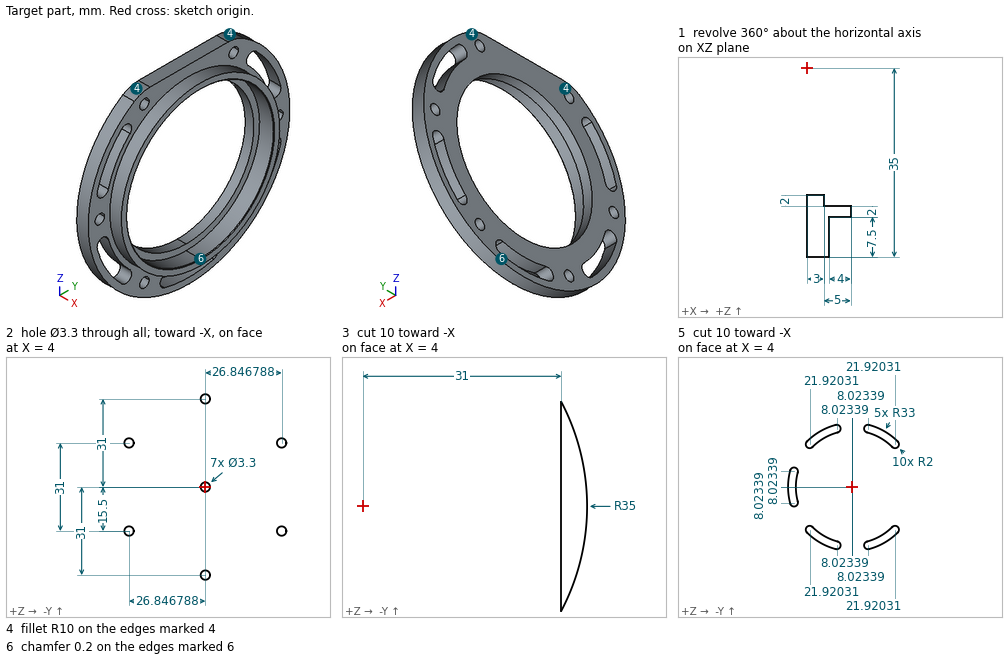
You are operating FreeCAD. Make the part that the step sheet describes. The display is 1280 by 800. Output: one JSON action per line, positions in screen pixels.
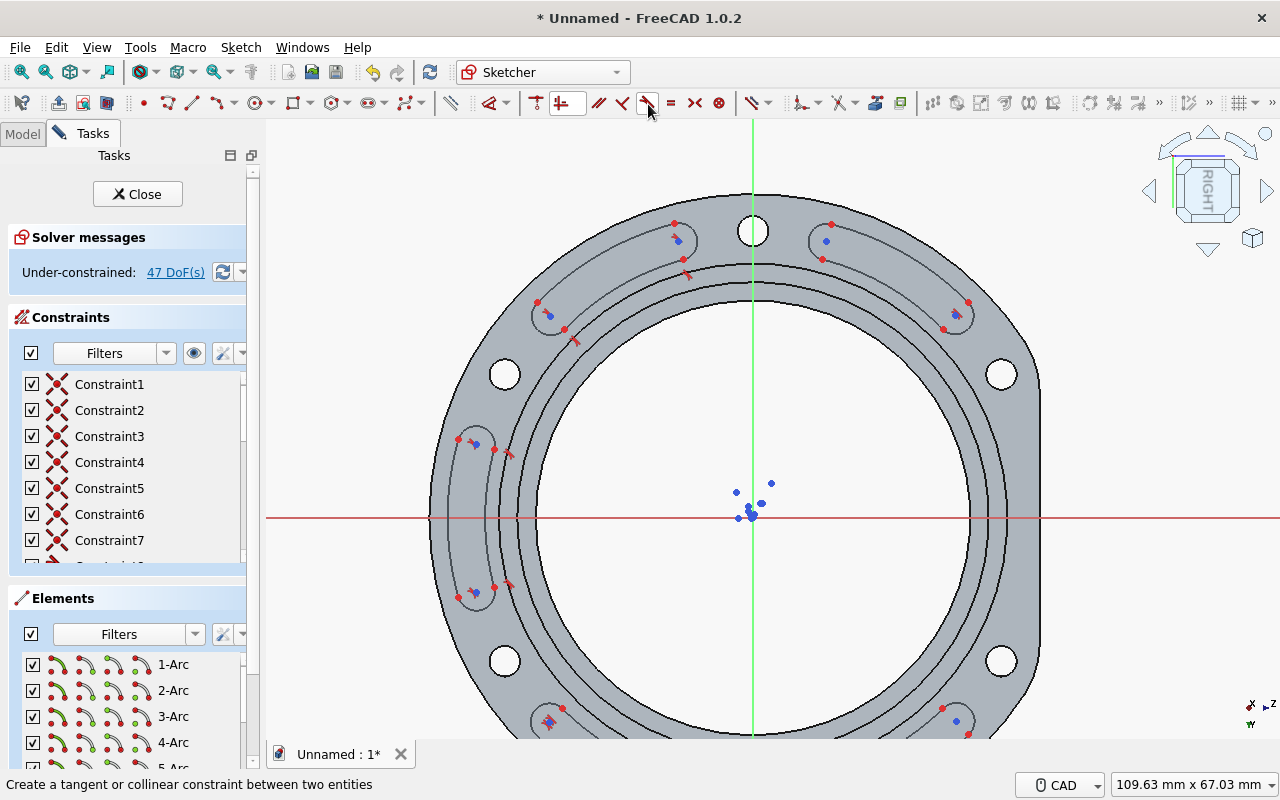
{"action": "left_click", "coordinate": [959, 334]}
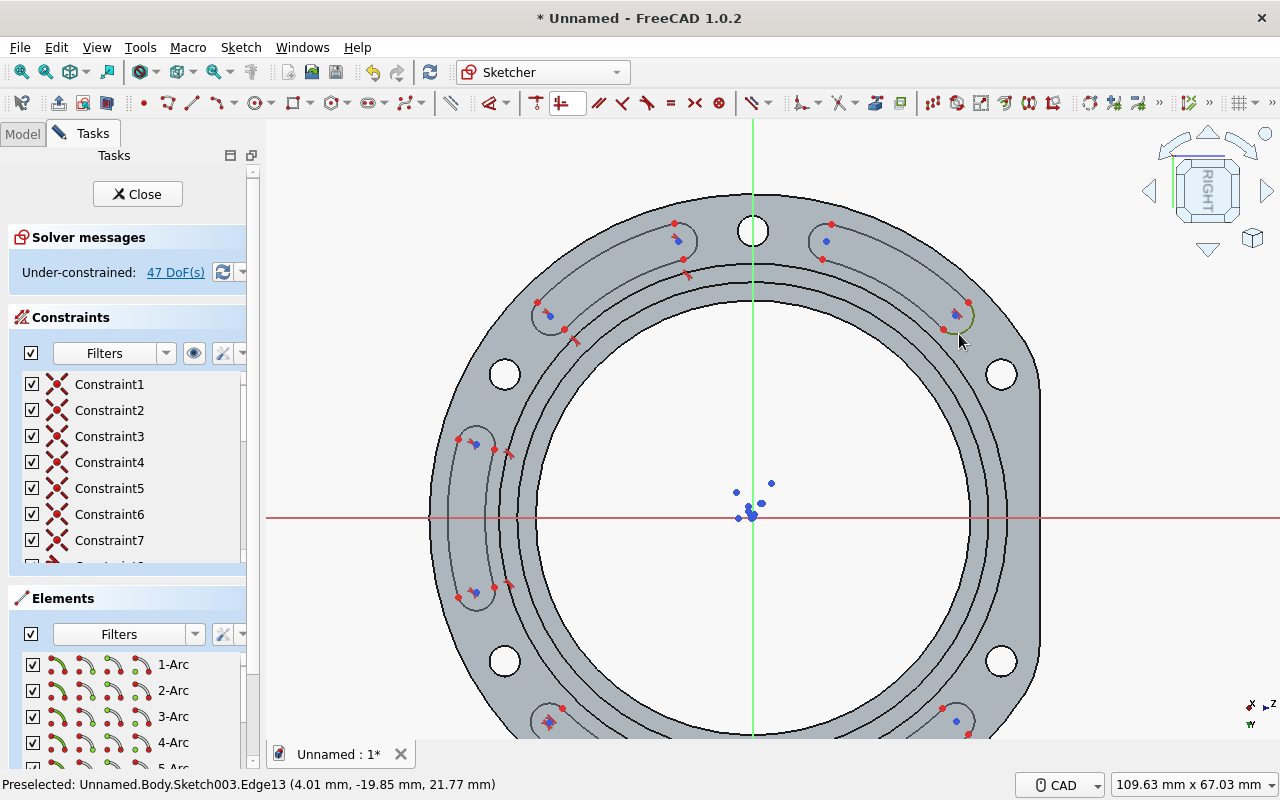
{"action": "left_click", "coordinate": [911, 302]}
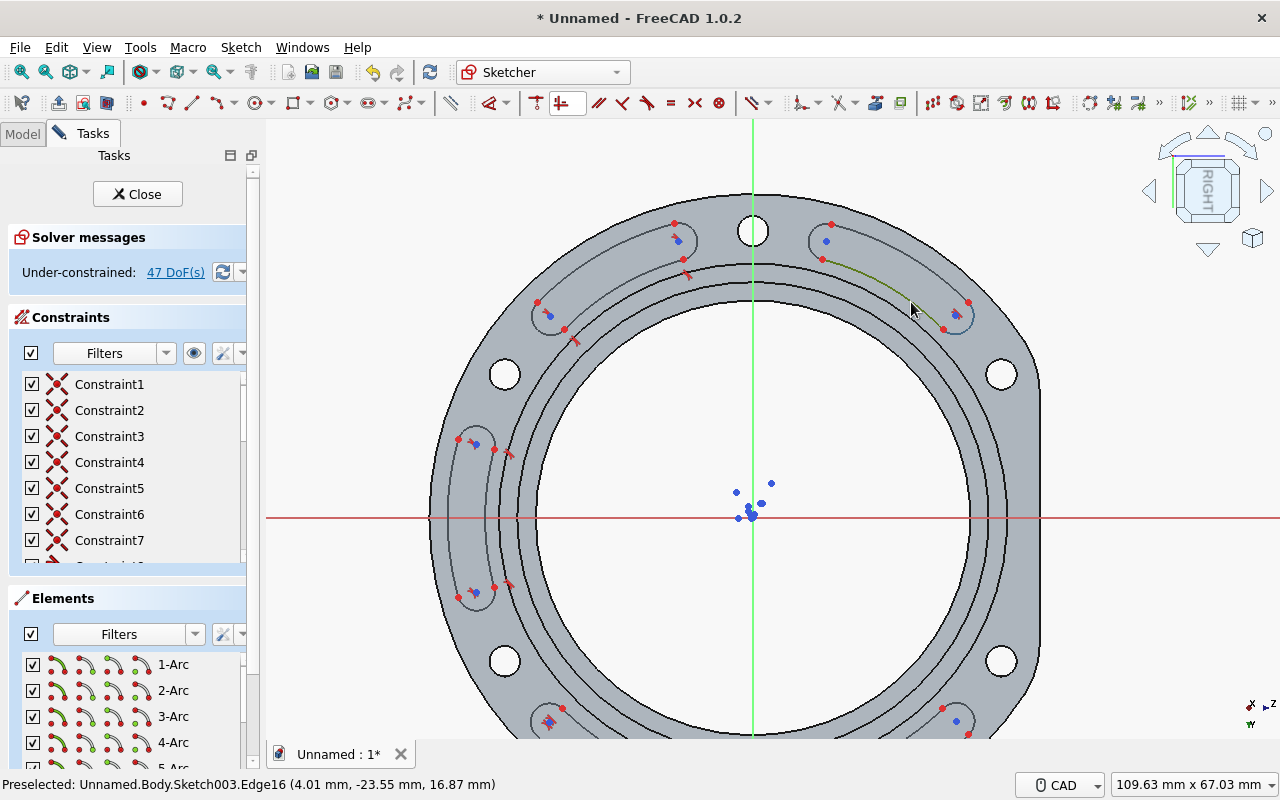
{"action": "left_click", "coordinate": [648, 104]}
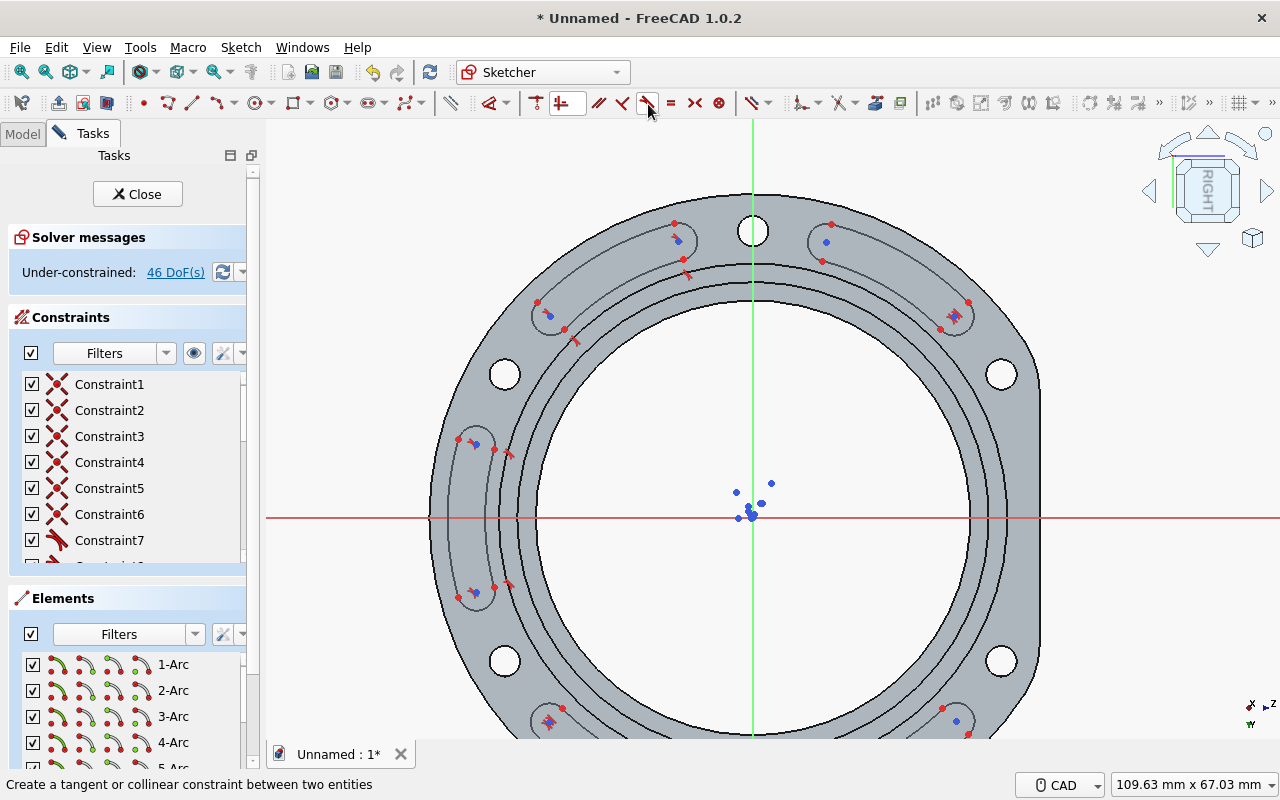
{"action": "left_click", "coordinate": [932, 272]}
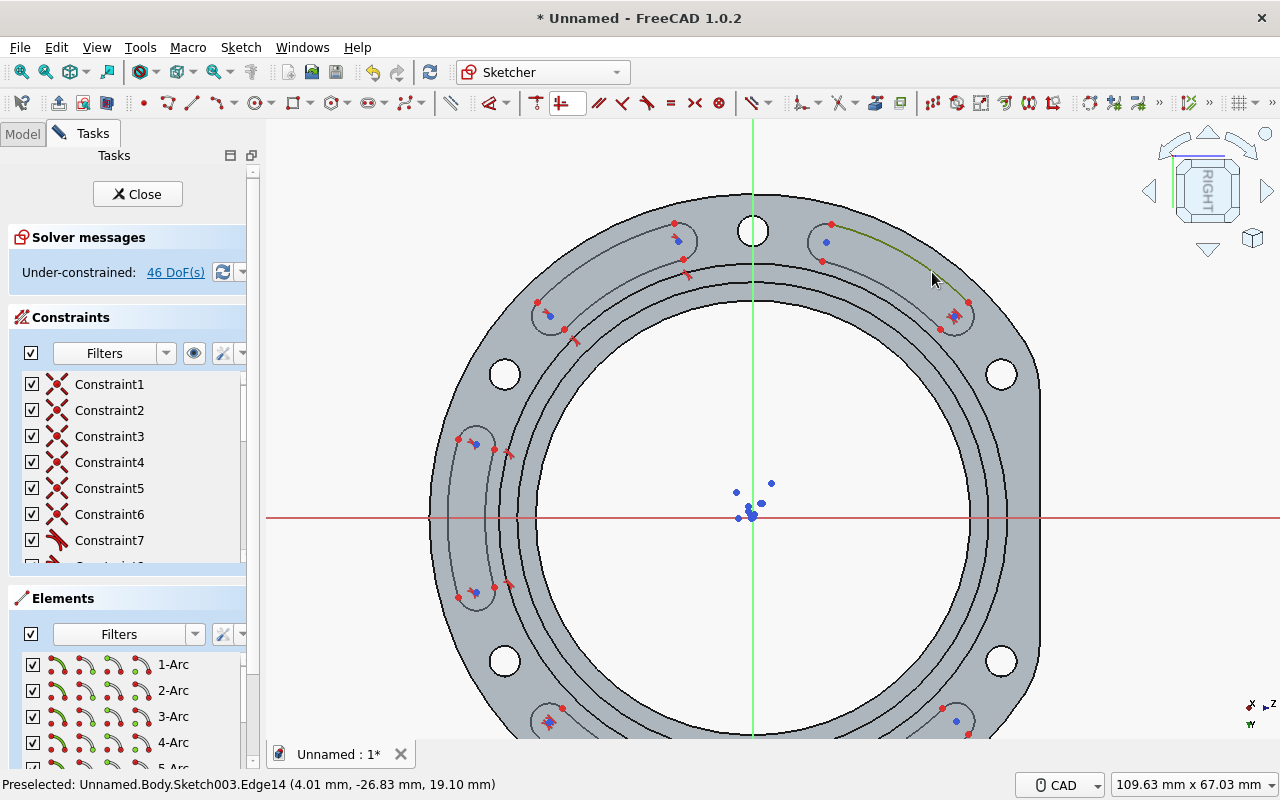
{"action": "left_click", "coordinate": [815, 228]}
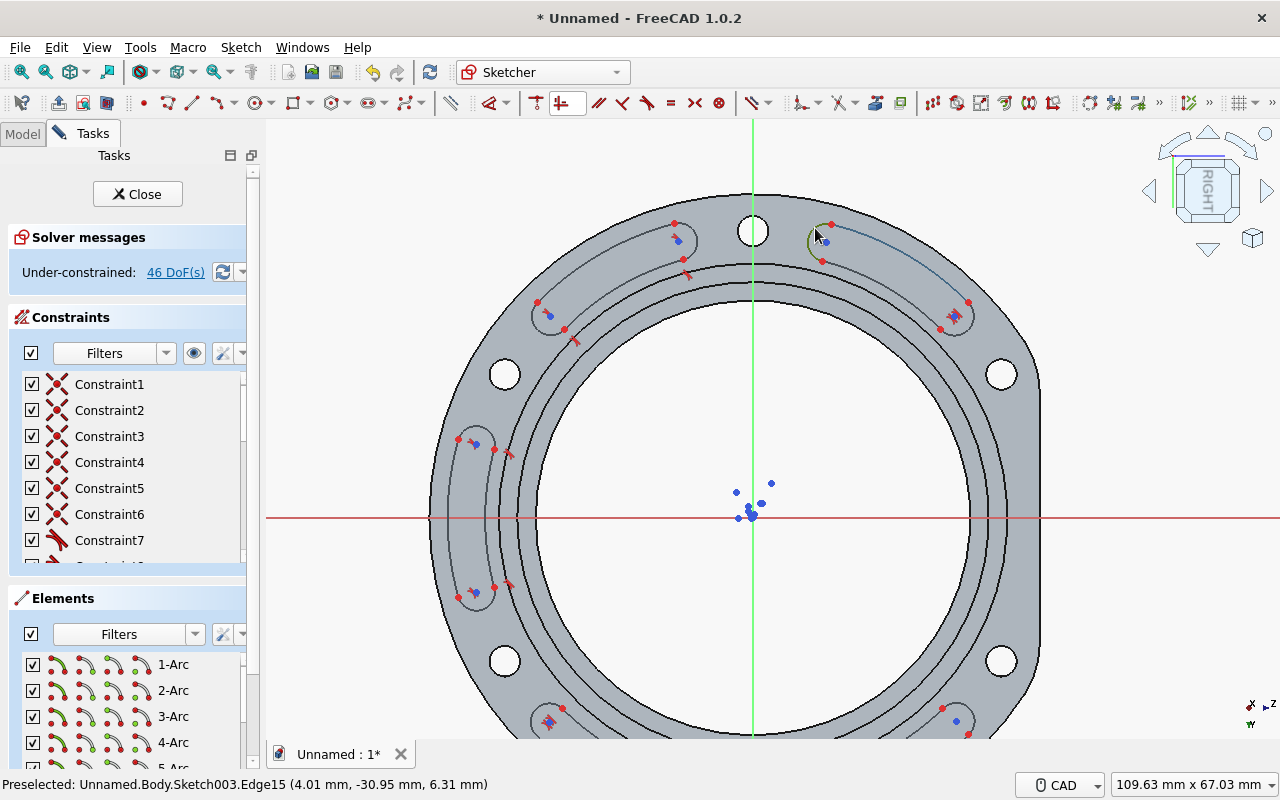
{"action": "left_click", "coordinate": [648, 104]}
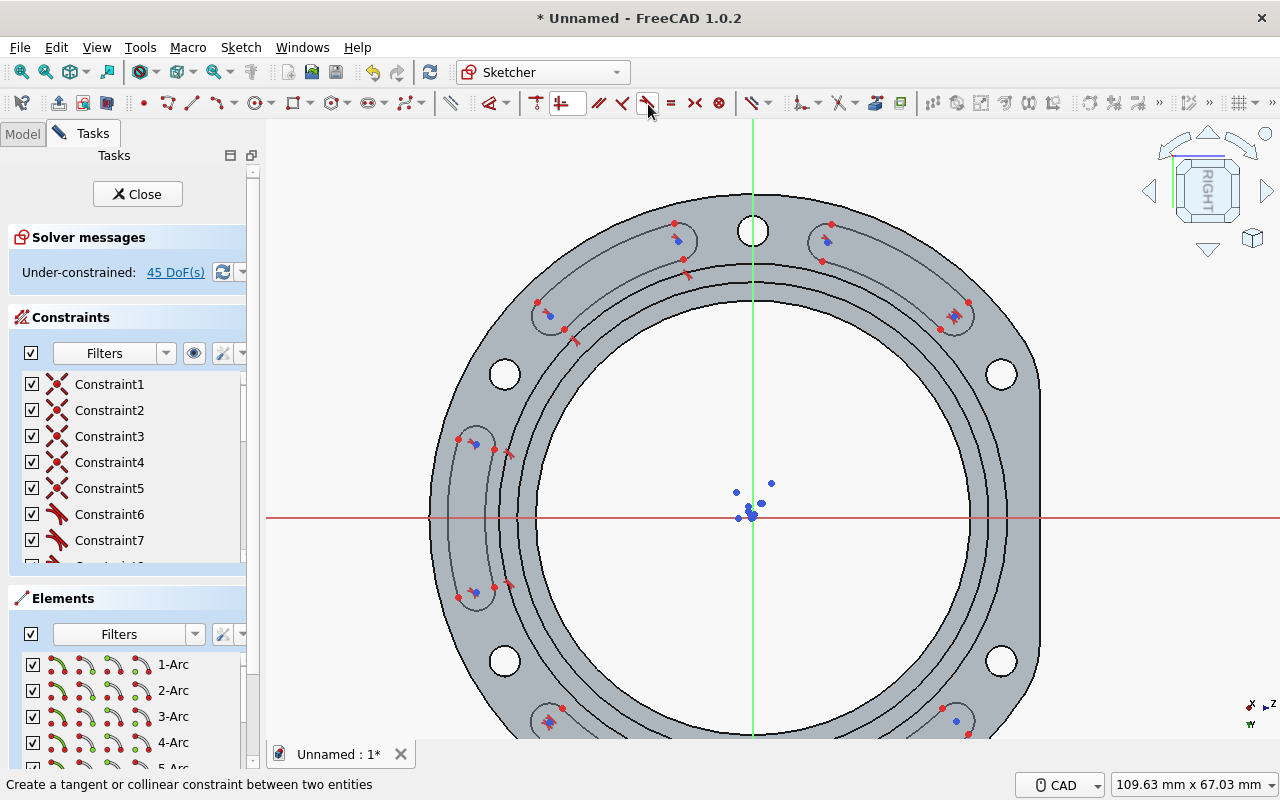
{"action": "left_click", "coordinate": [815, 228]}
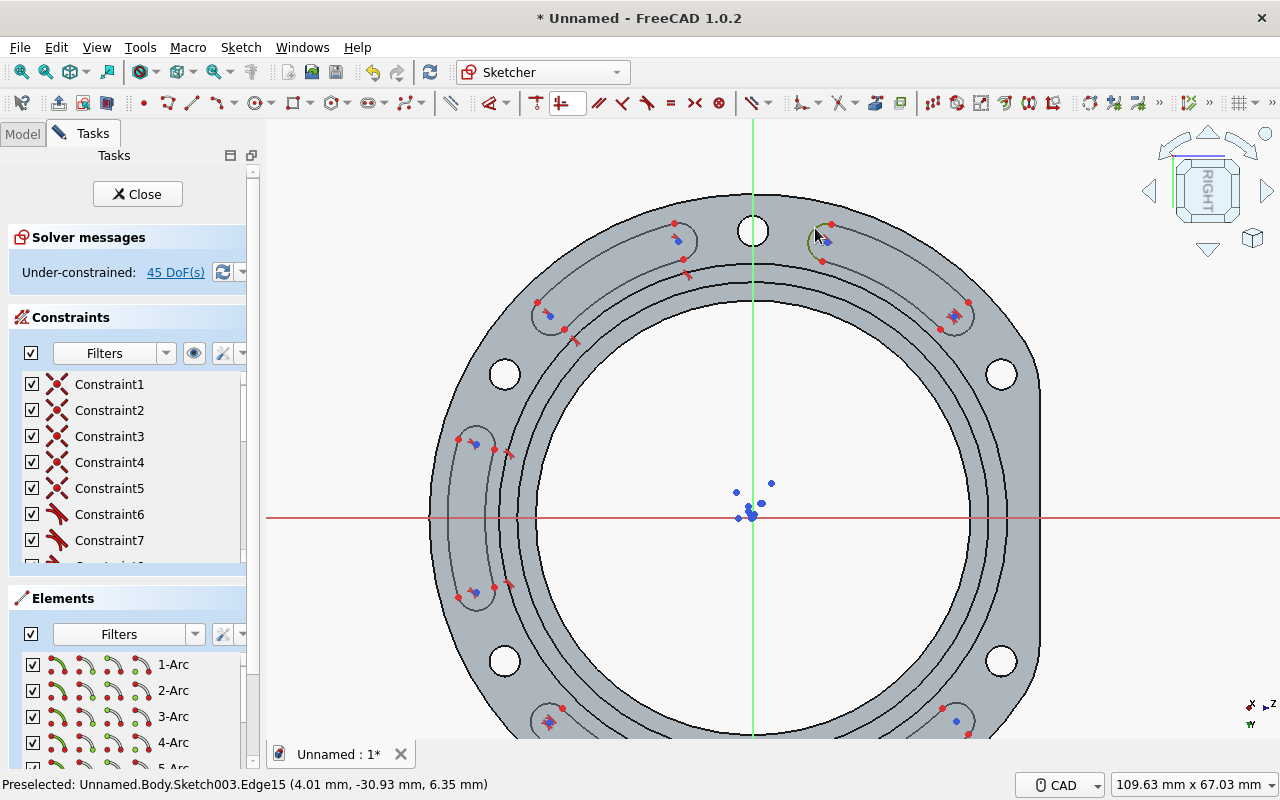
{"action": "left_click", "coordinate": [910, 302]}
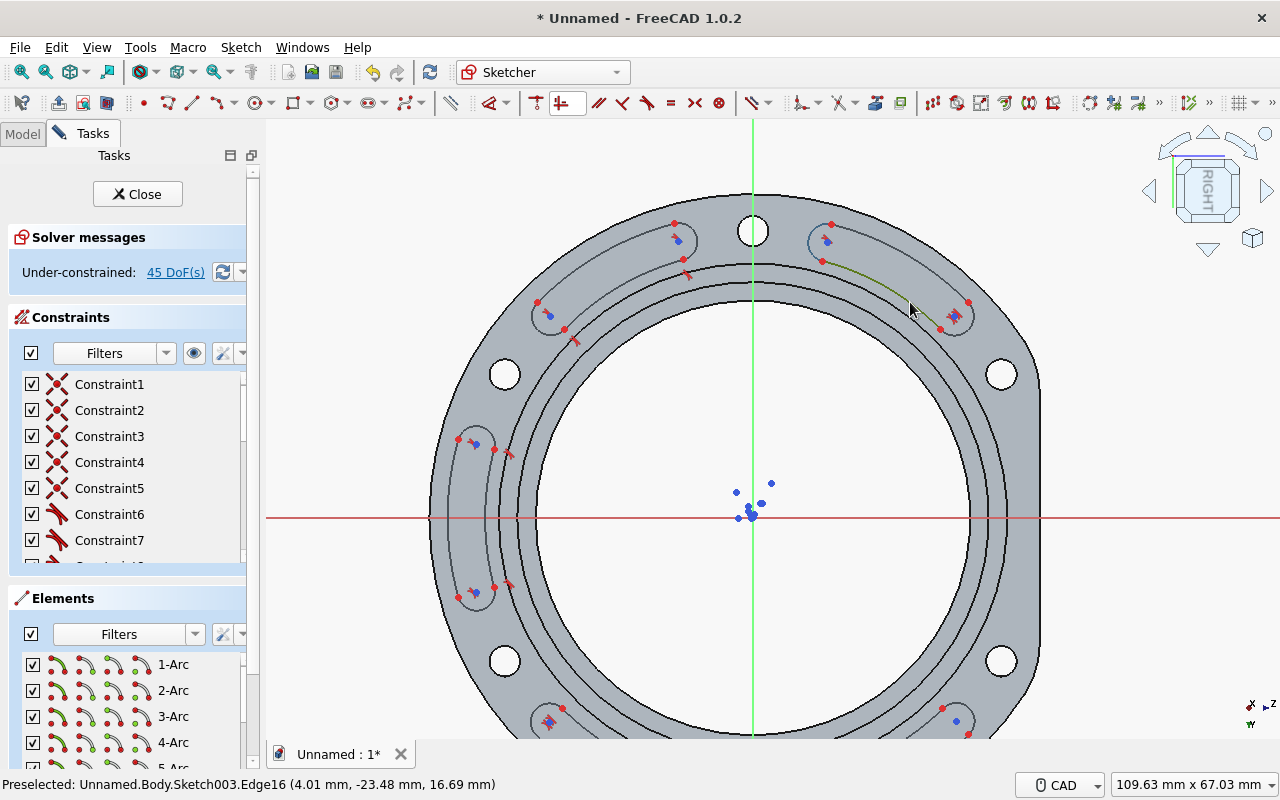
{"action": "left_click", "coordinate": [648, 104]}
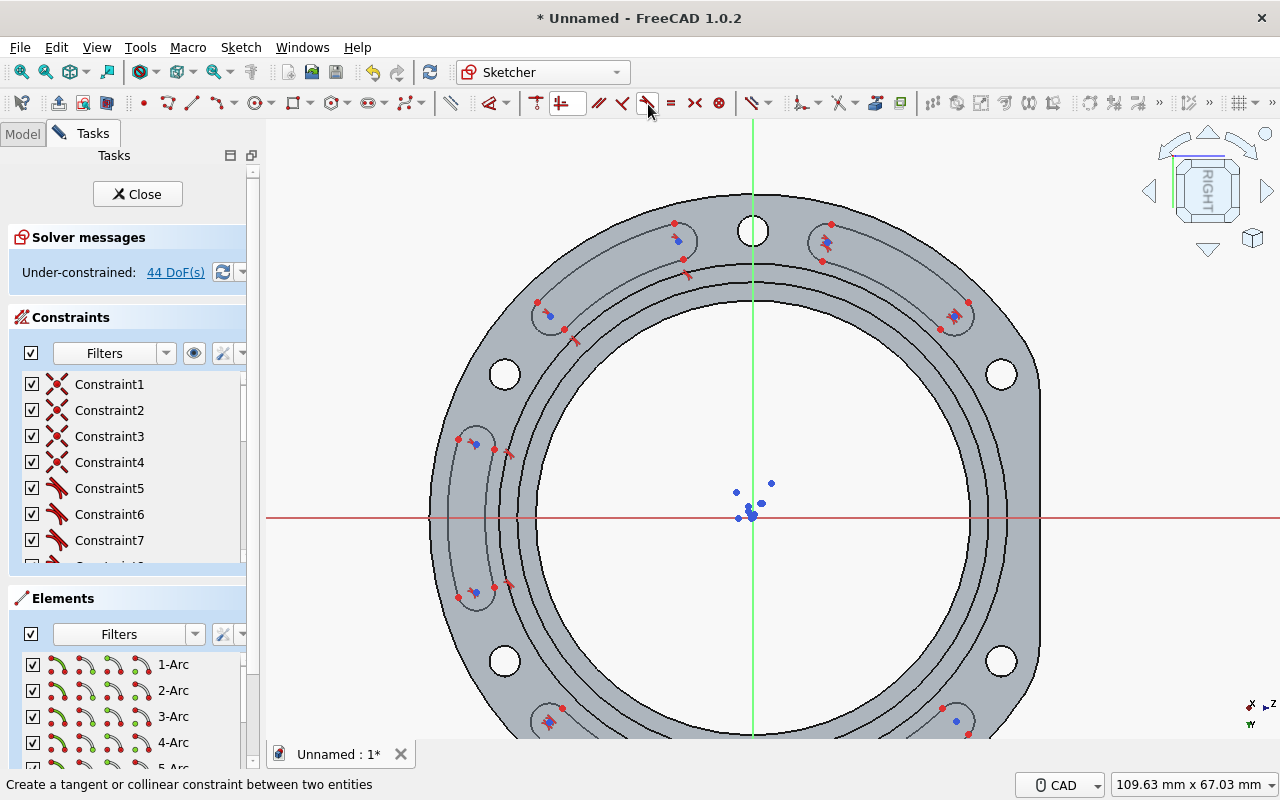
{"action": "scroll", "coordinate": [697, 248], "scroll_direction": "down", "scroll_amount": 2}